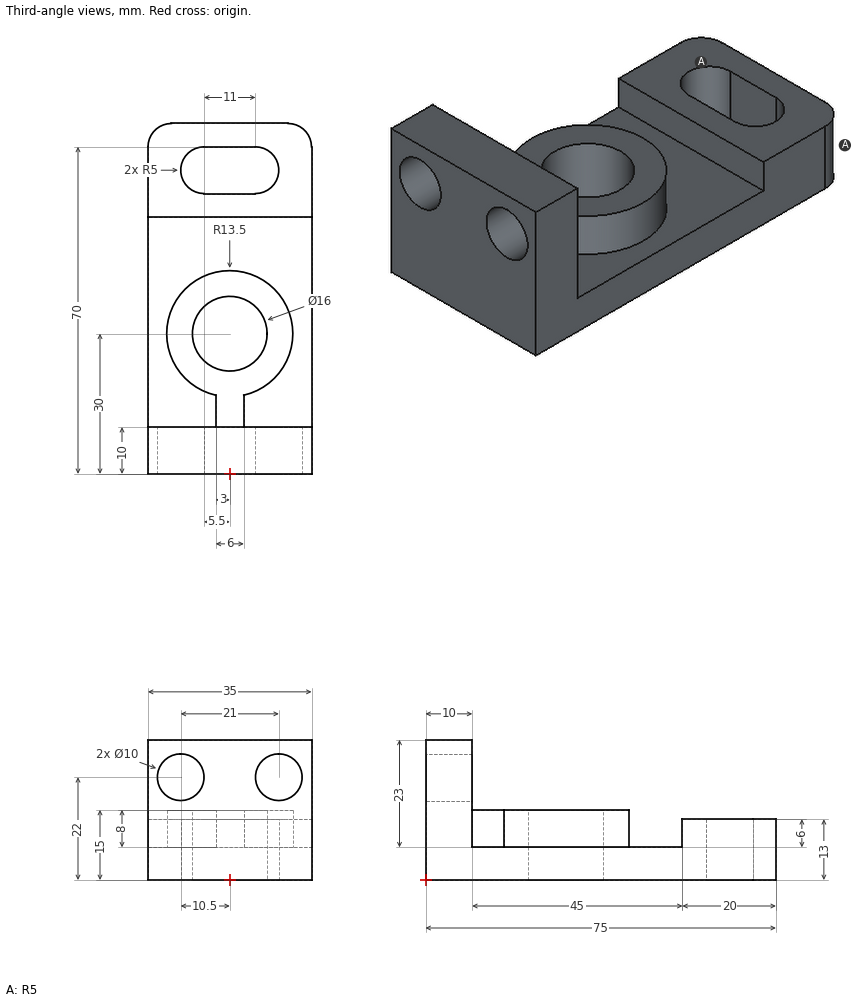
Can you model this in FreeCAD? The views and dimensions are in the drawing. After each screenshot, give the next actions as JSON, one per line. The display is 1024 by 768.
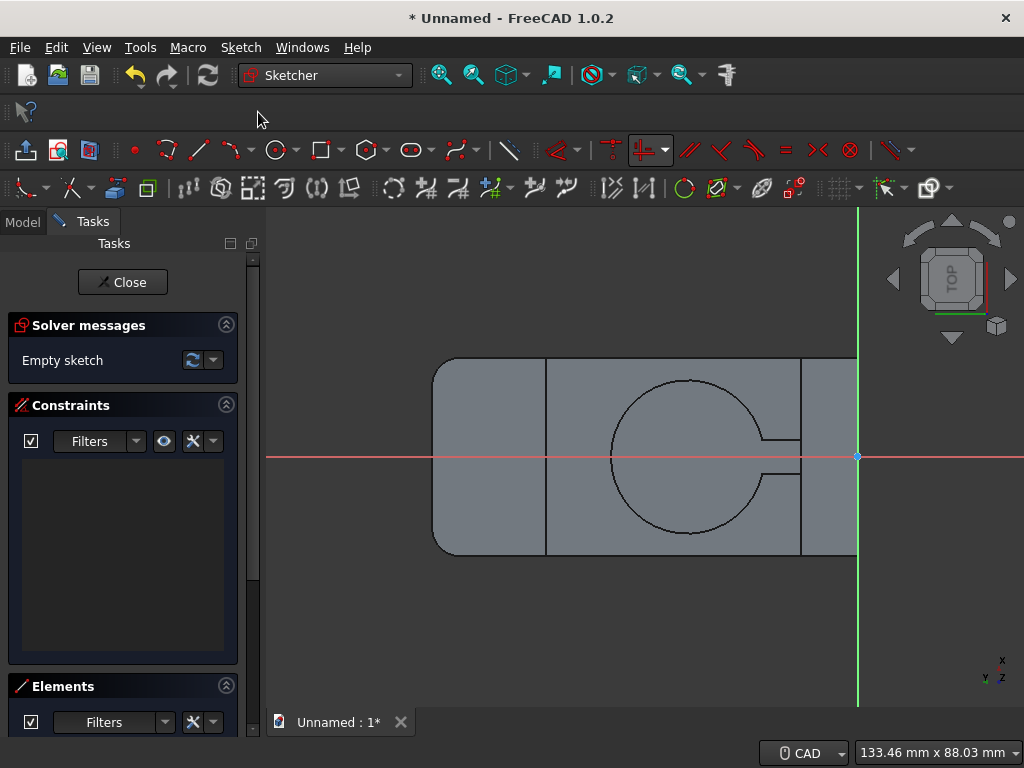
{"action": "scroll", "coordinate": [294, 457], "scroll_direction": "down", "scroll_amount": 1}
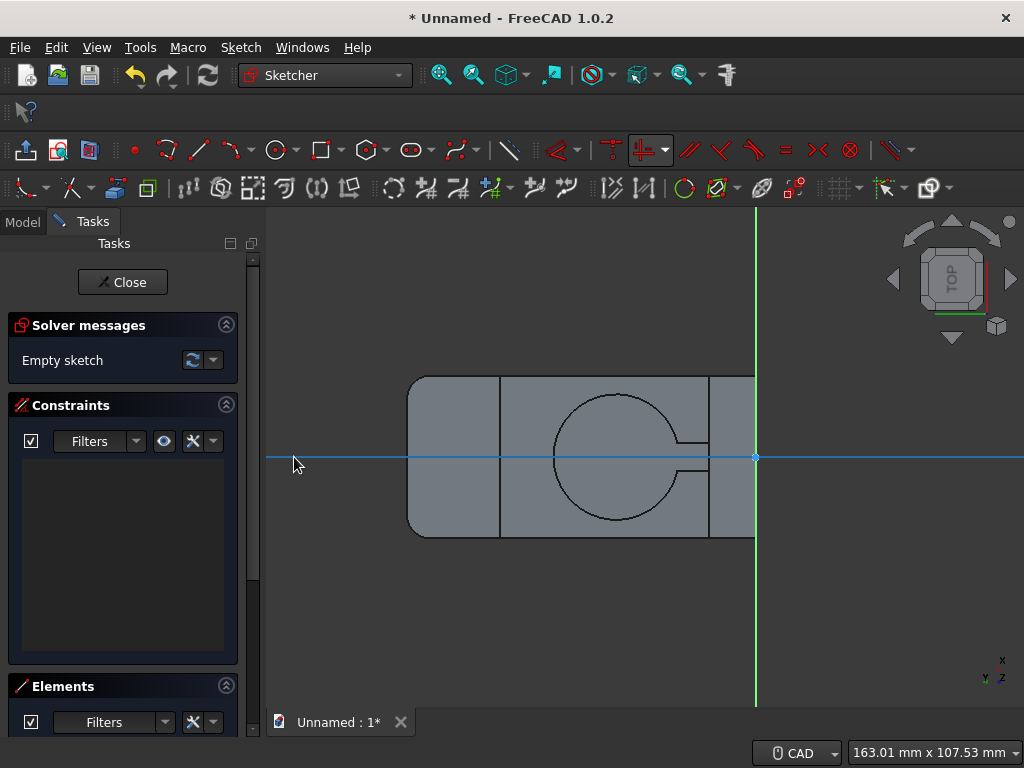
{"action": "key", "text": "g s"}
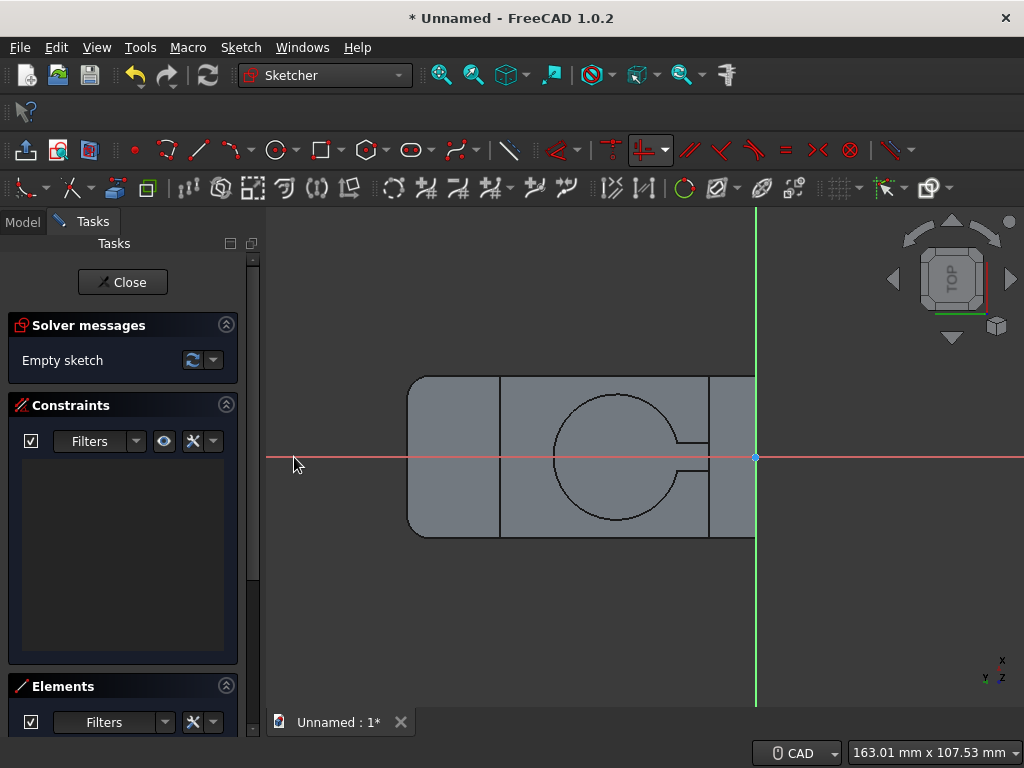
{"action": "left_click", "coordinate": [454, 483]}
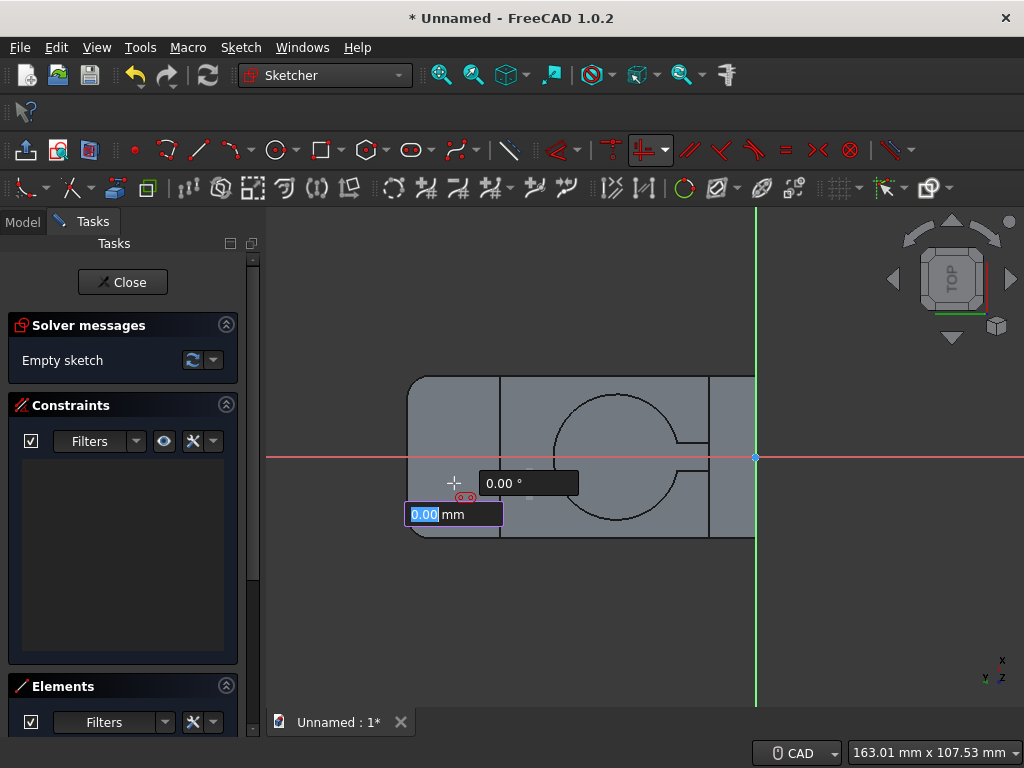
{"action": "left_click", "coordinate": [454, 432]}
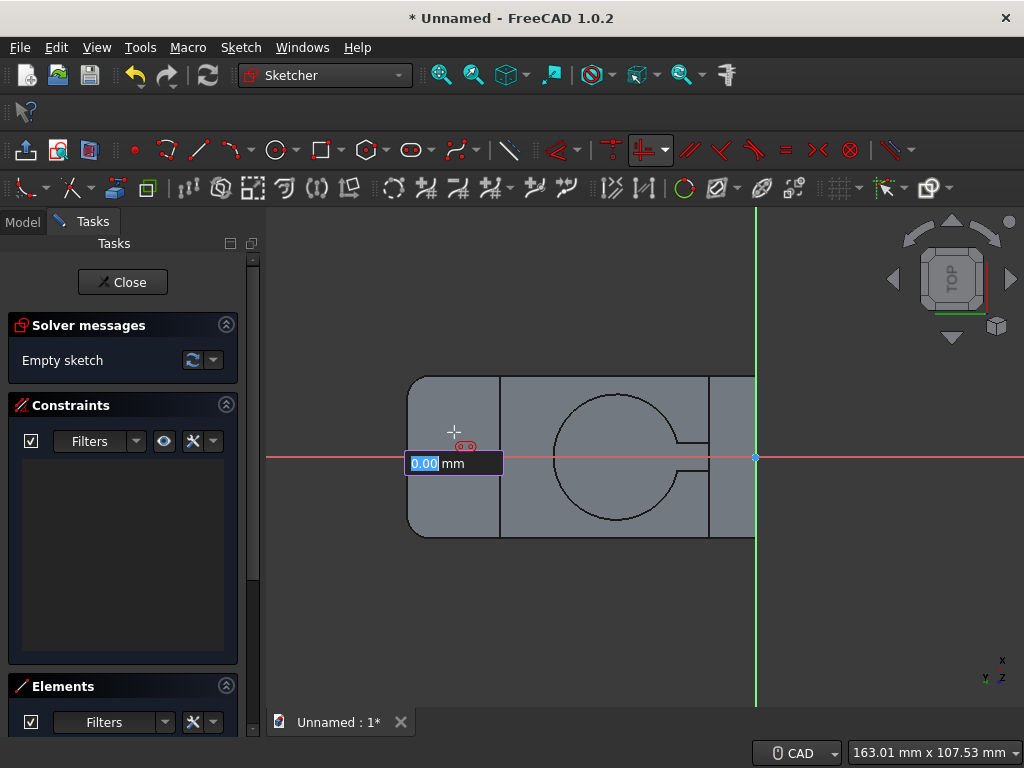
{"action": "scroll", "coordinate": [430, 449], "scroll_direction": "up", "scroll_amount": 4}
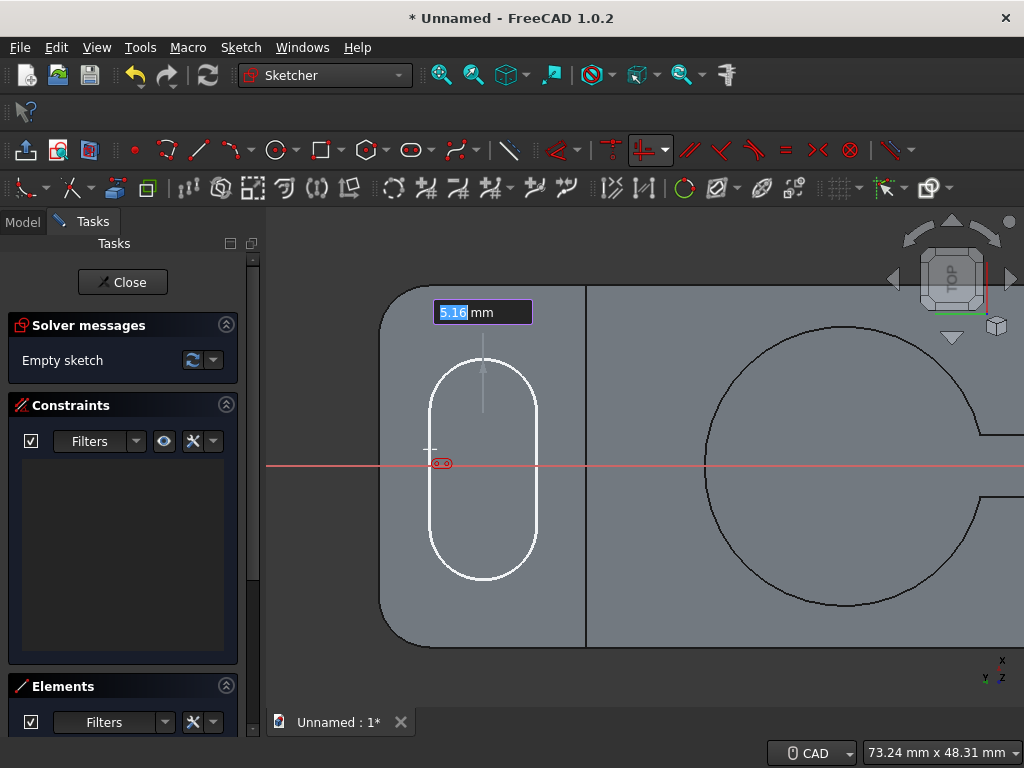
{"action": "left_click", "coordinate": [430, 449]}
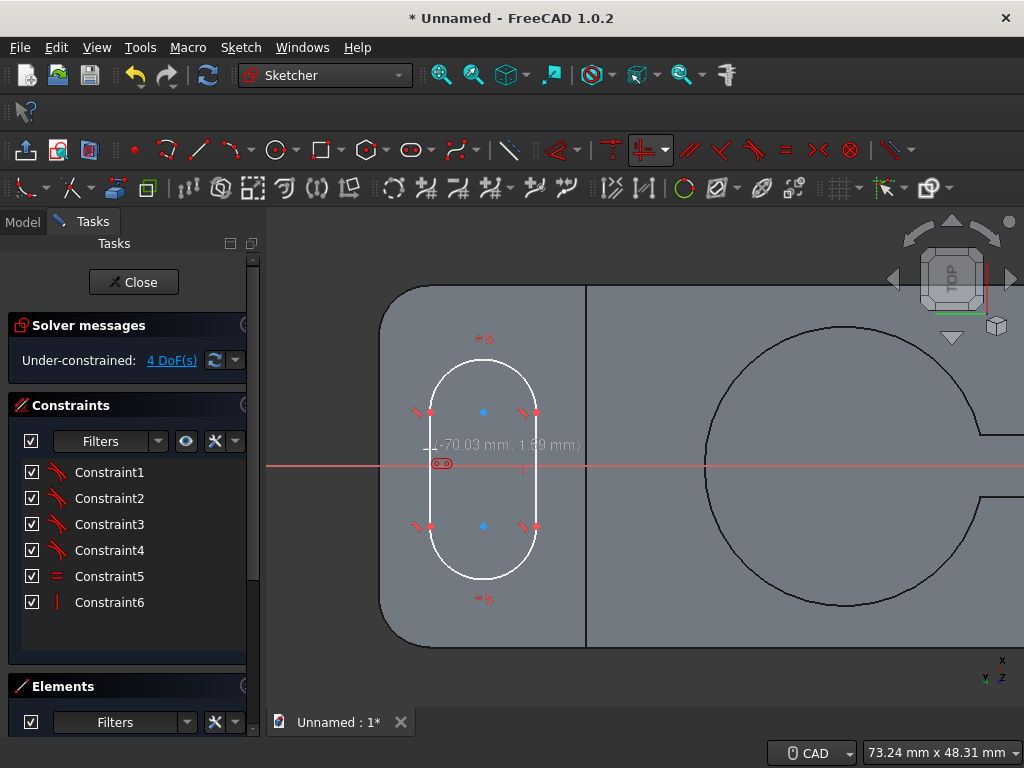
{"action": "left_click", "coordinate": [276, 150]}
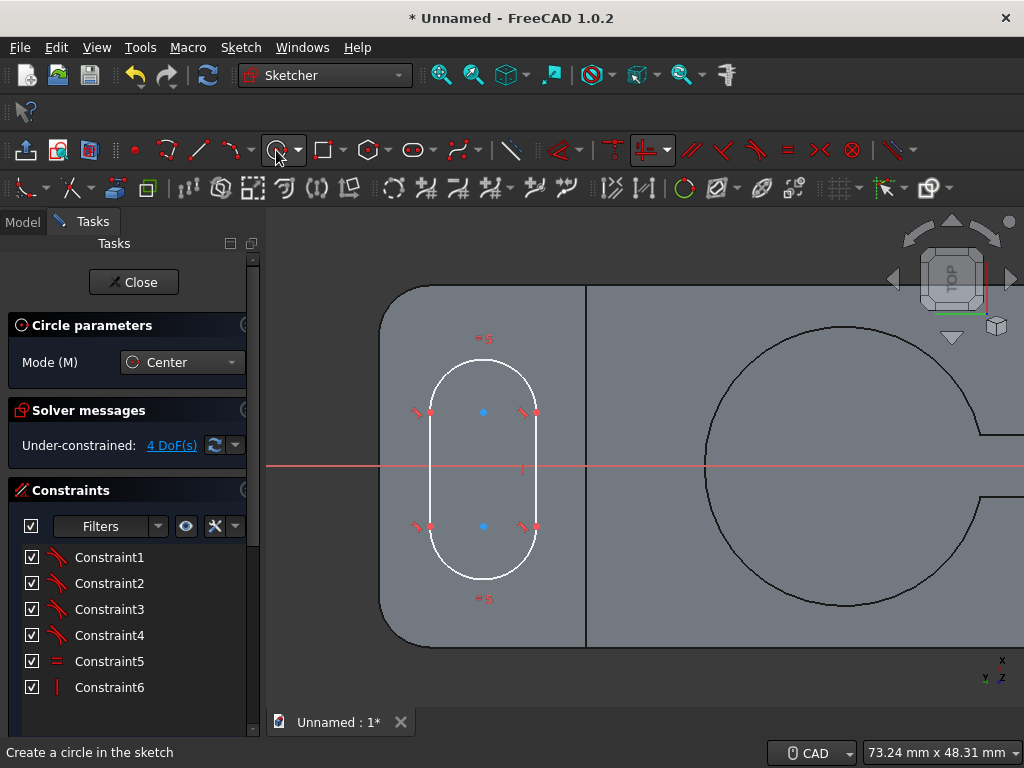
{"action": "left_click", "coordinate": [844, 466]}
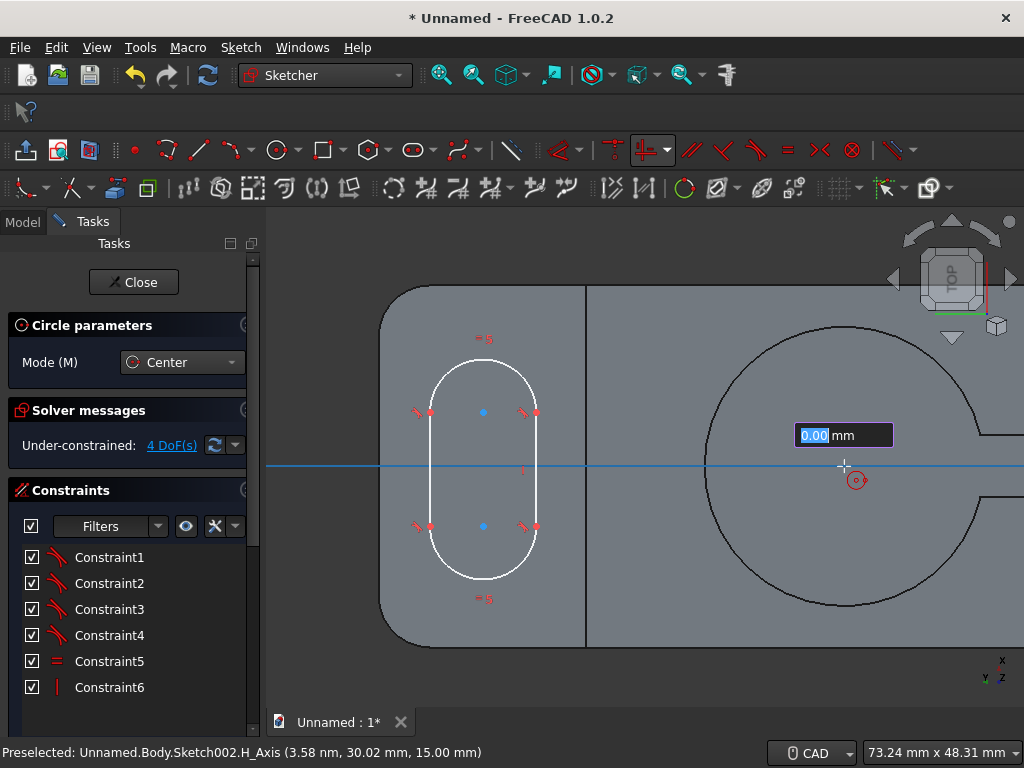
{"action": "scroll", "coordinate": [314, 446], "scroll_direction": "down", "scroll_amount": 3}
{"action": "mouse_move", "coordinate": [637, 425]}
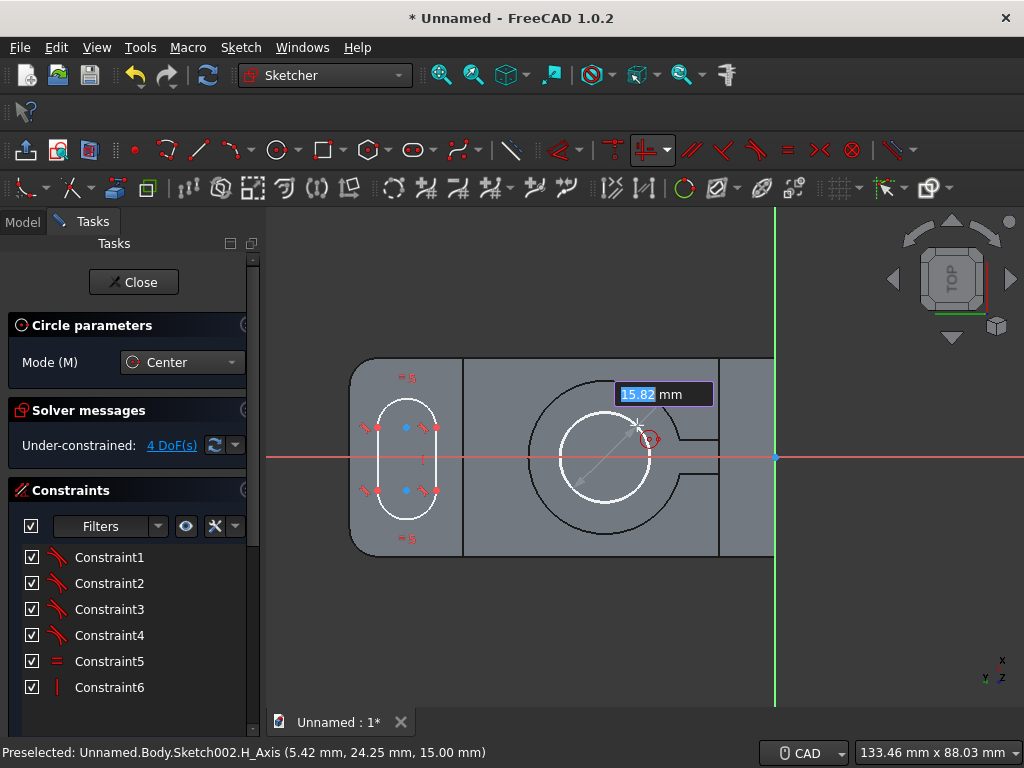
{"action": "type", "text": "16"}
{"action": "key", "text": "Return"}
{"action": "key", "text": "Escape"}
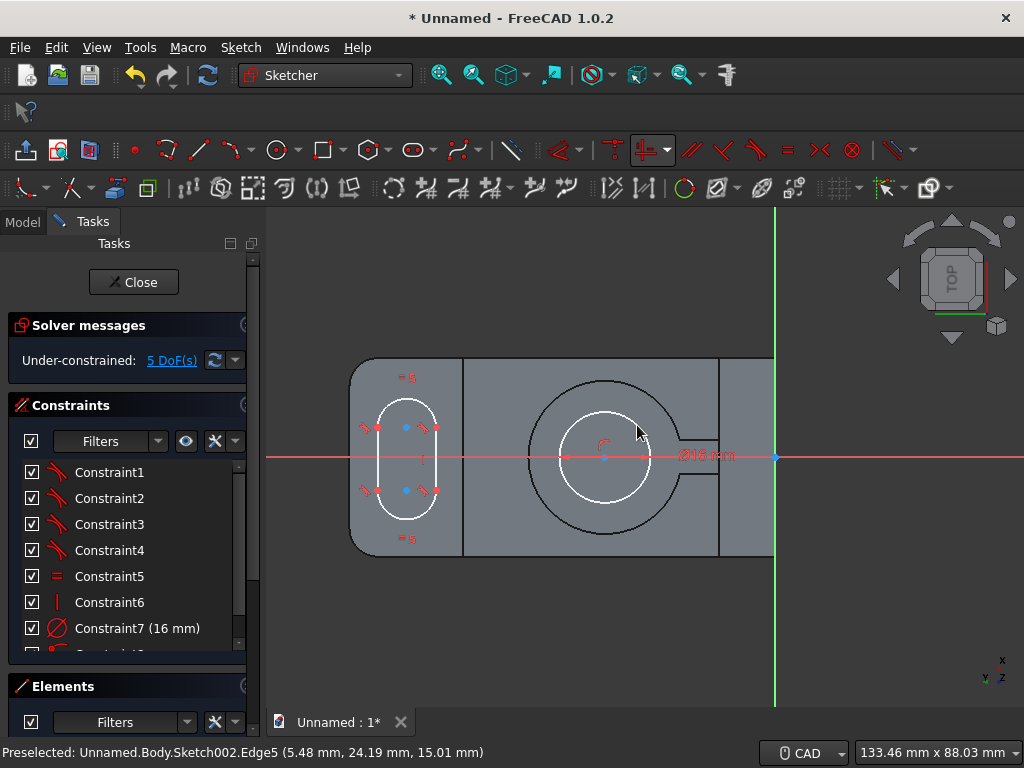
{"action": "key", "text": "d"}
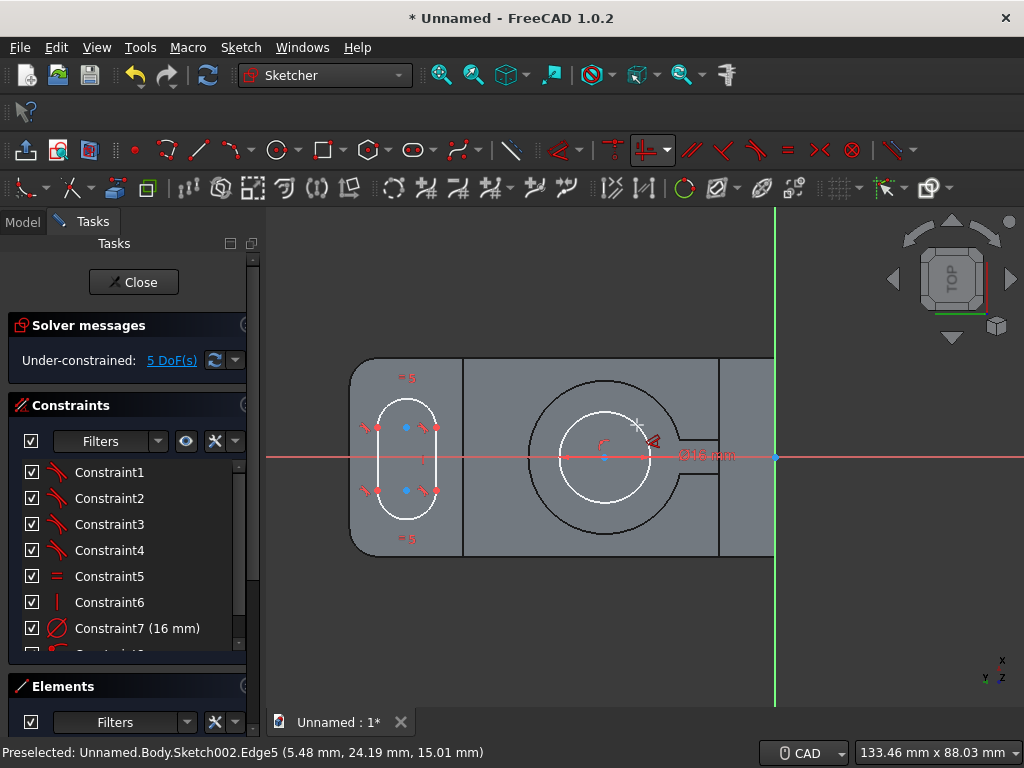
{"action": "scroll", "coordinate": [390, 514], "scroll_direction": "up", "scroll_amount": 2}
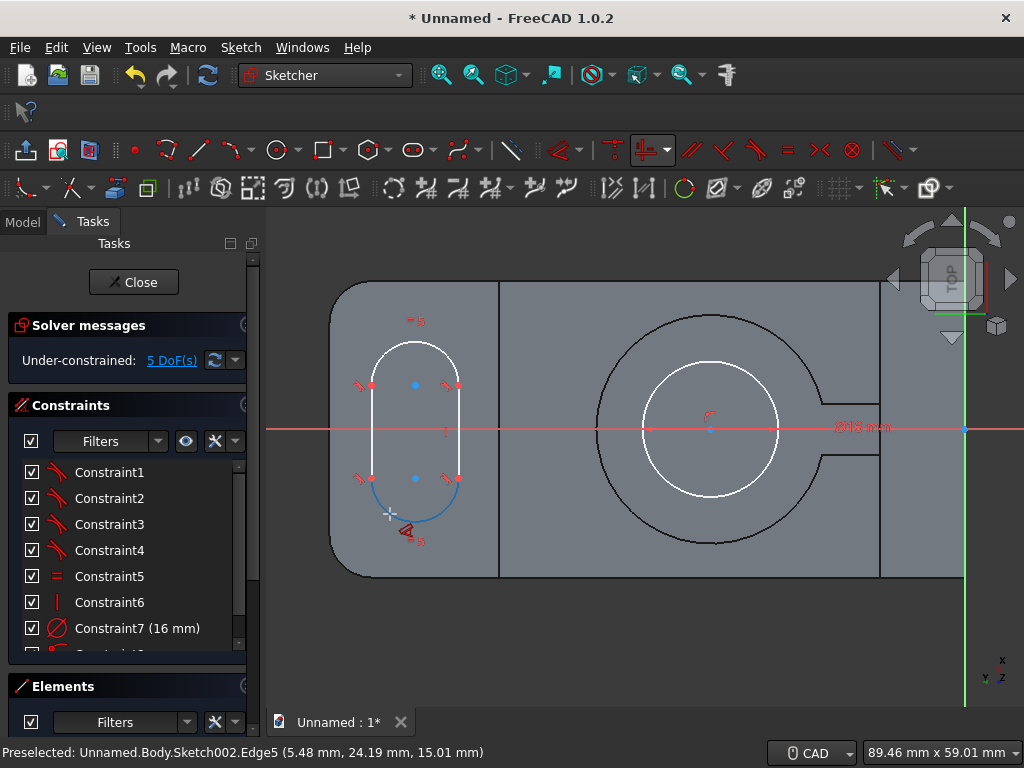
{"action": "left_click", "coordinate": [389, 514]}
{"action": "left_click", "coordinate": [370, 540]}